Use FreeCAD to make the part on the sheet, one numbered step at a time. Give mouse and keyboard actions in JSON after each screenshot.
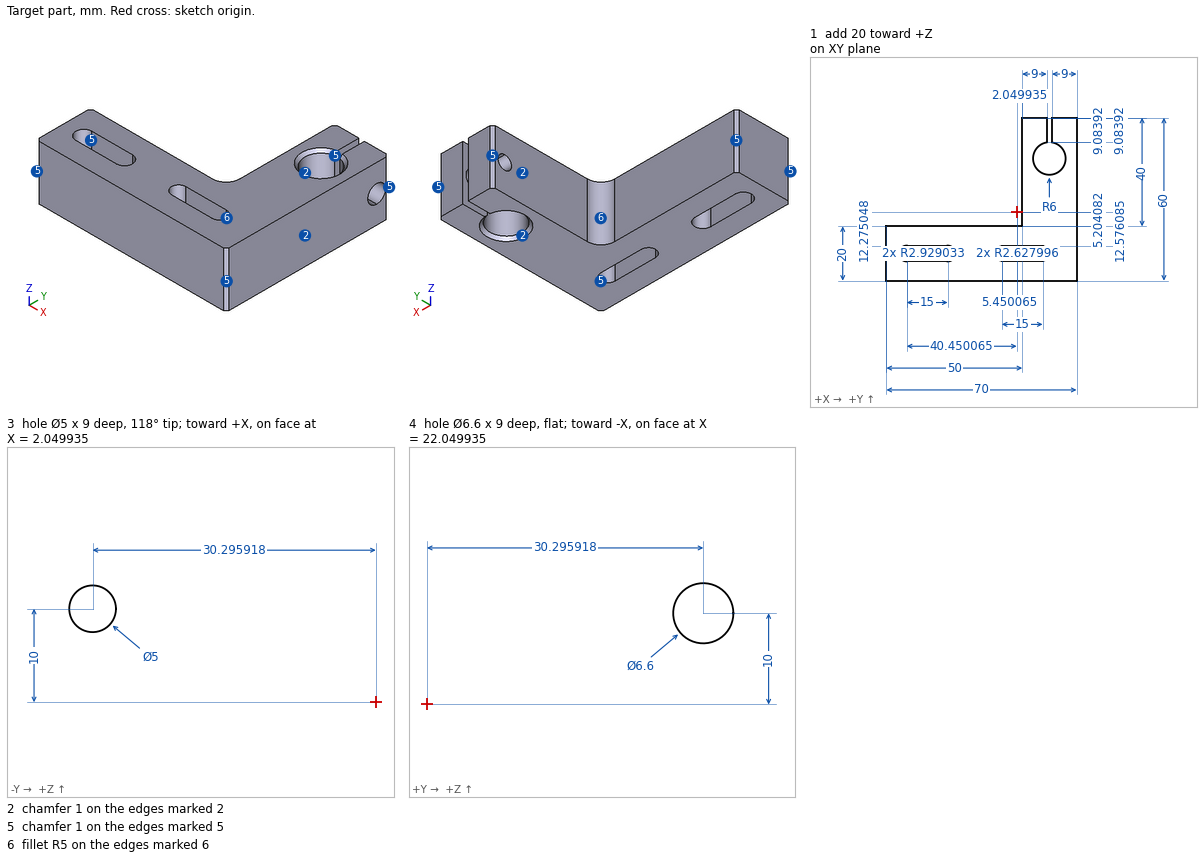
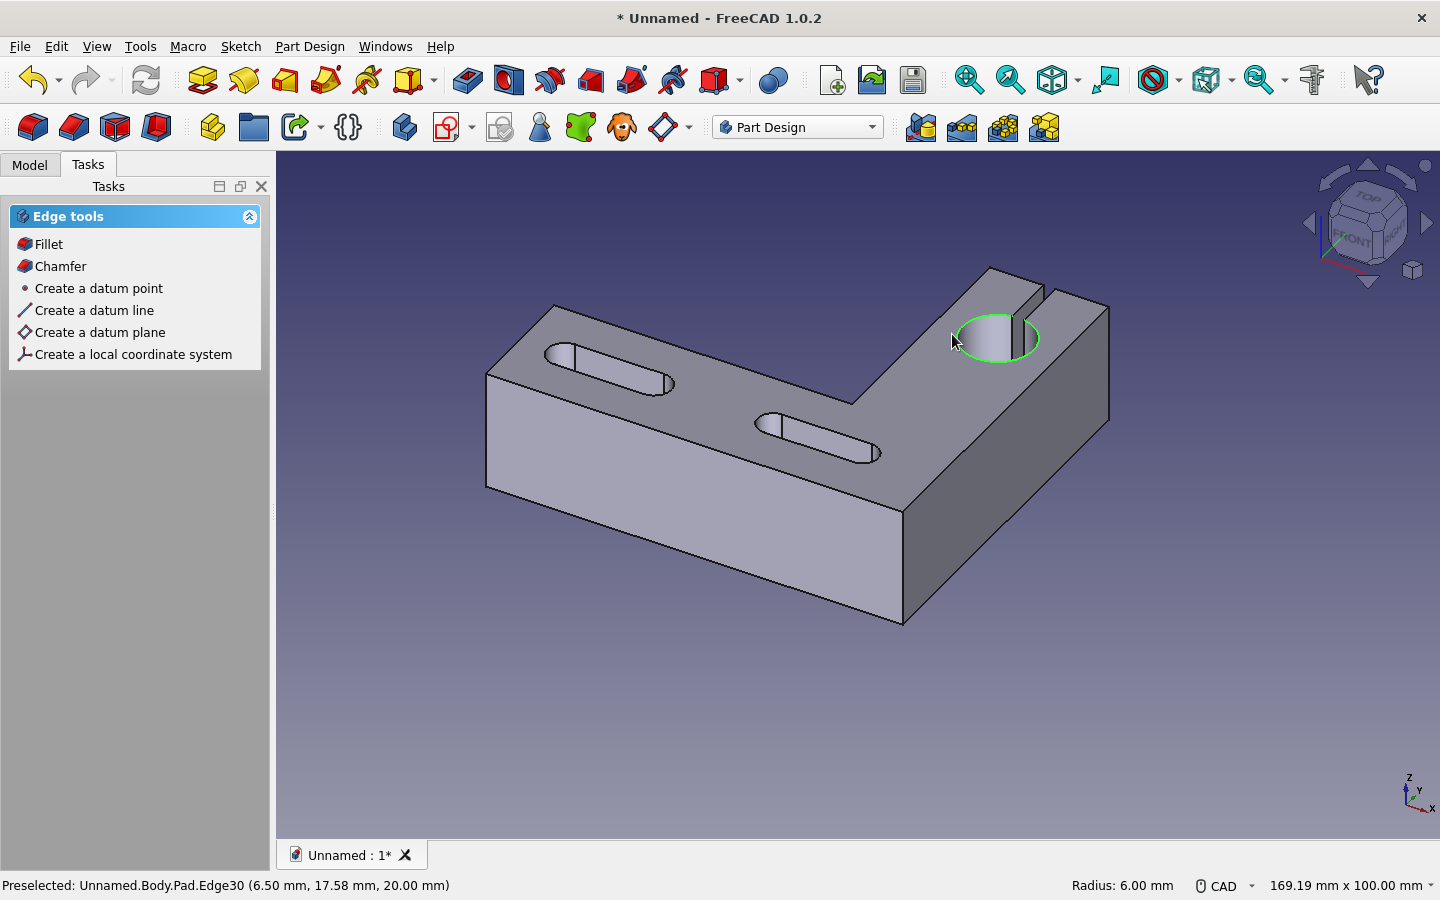
{"action": "key", "text": "0"}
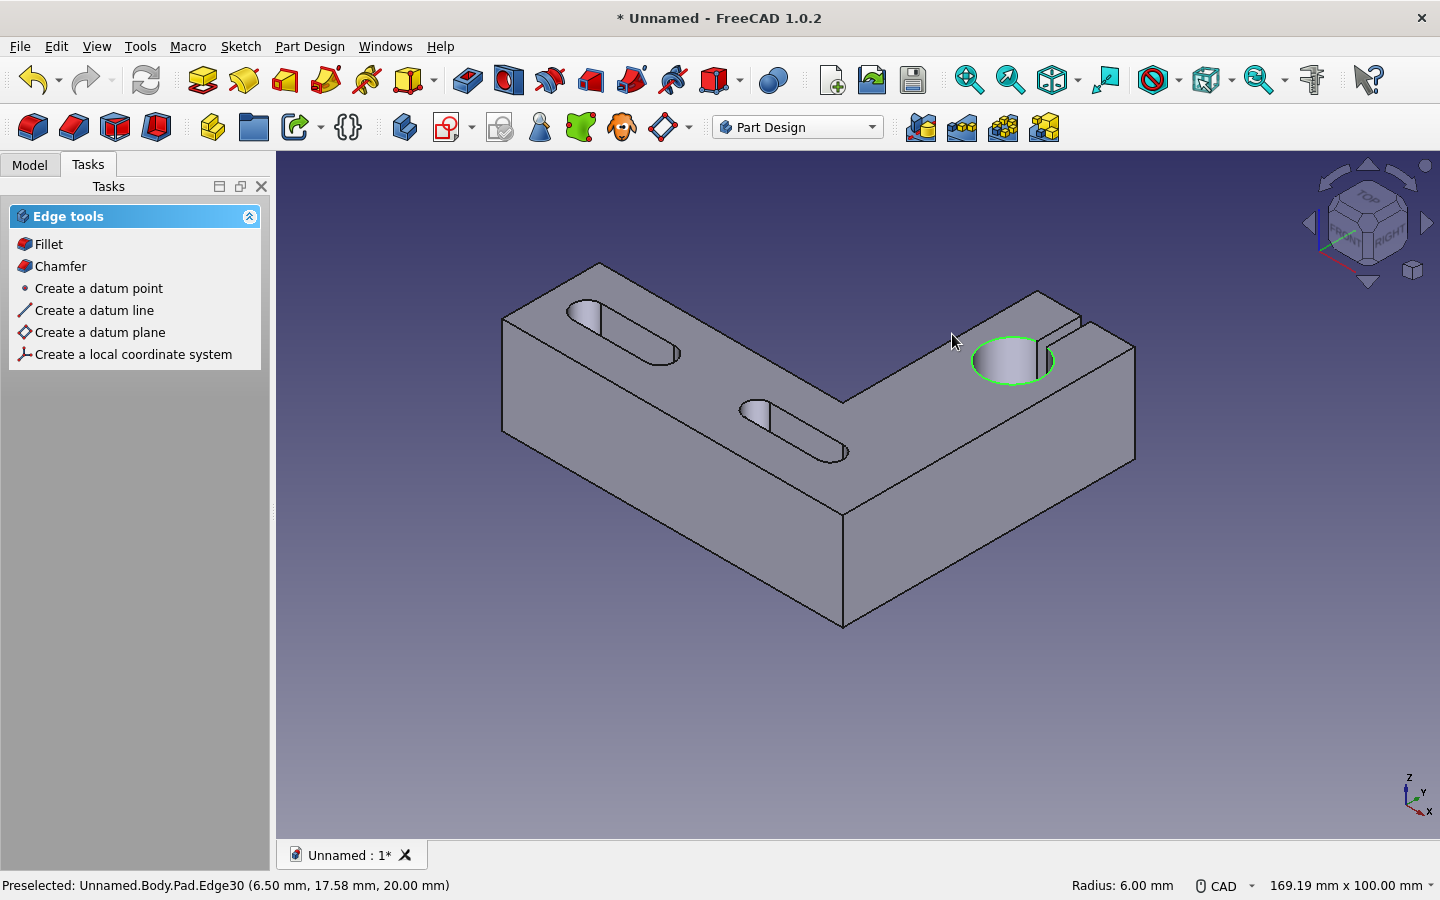
{"action": "left_click", "coordinate": [970, 80]}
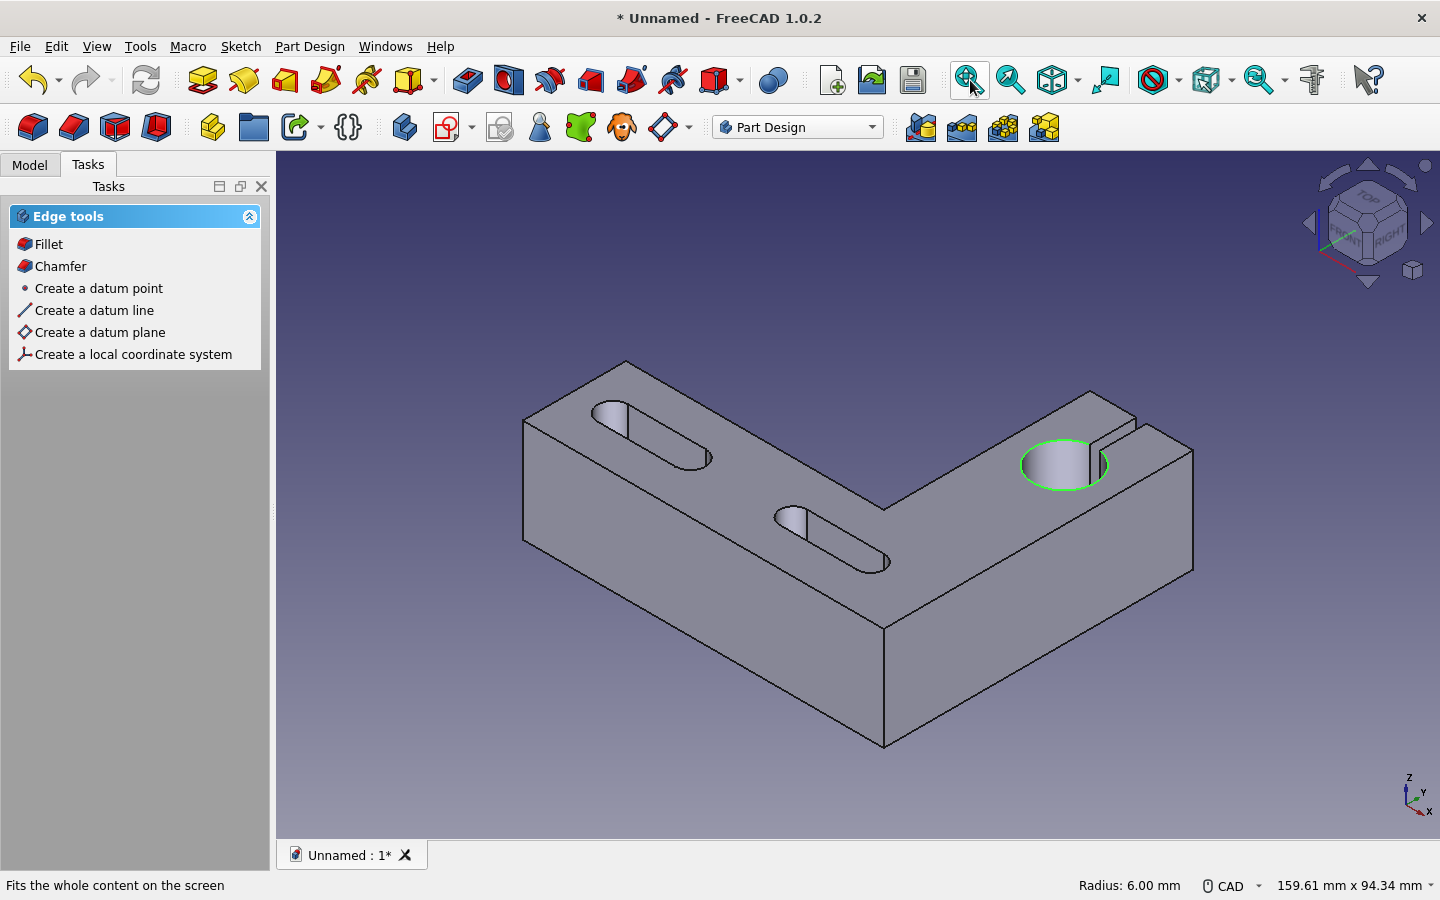
{"action": "key", "text": "2"}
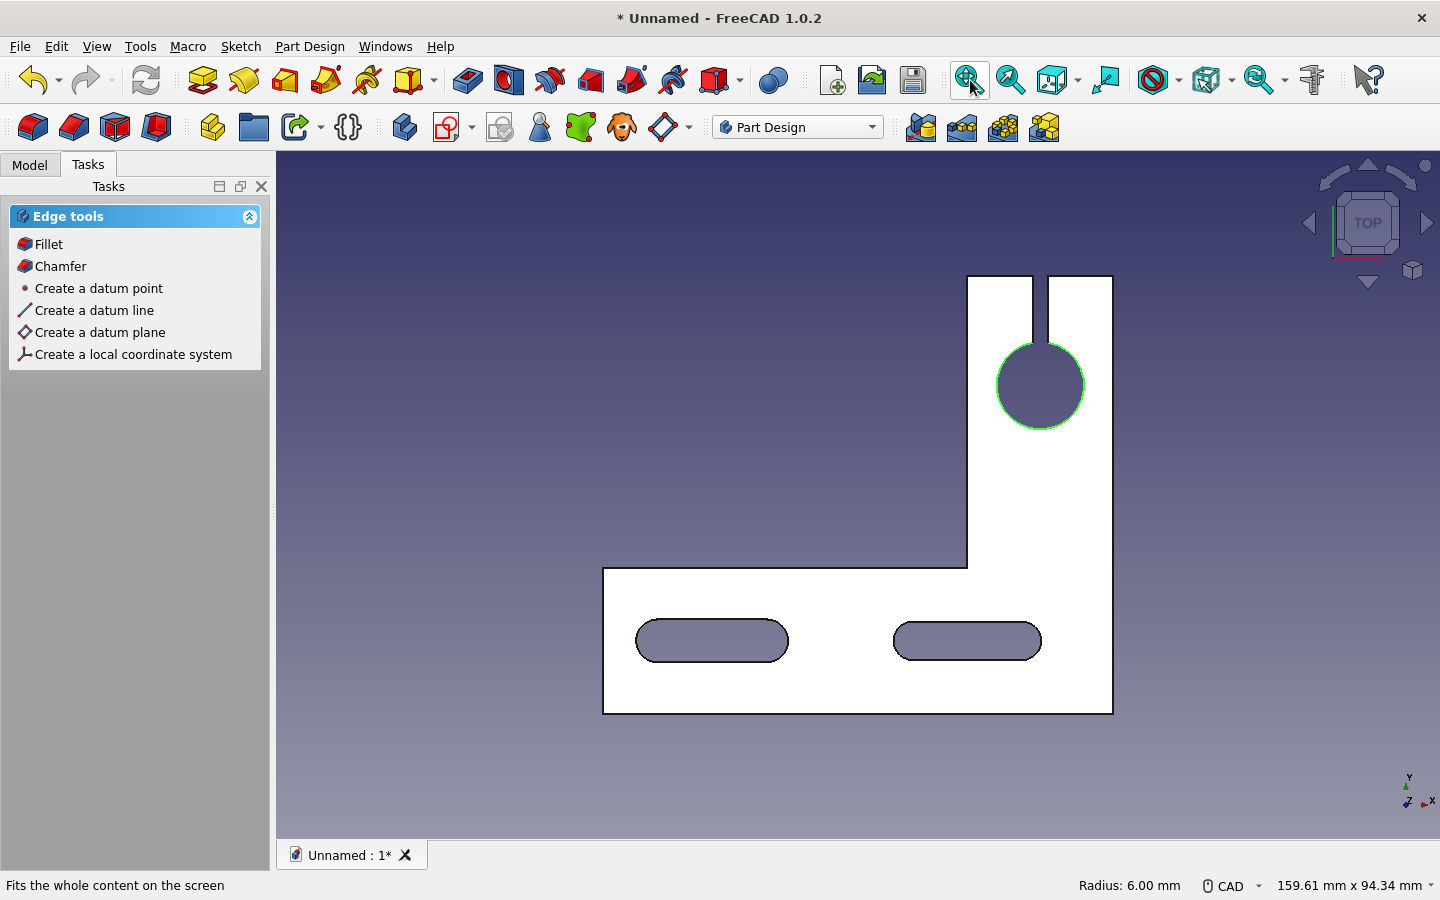
{"action": "key", "text": "1"}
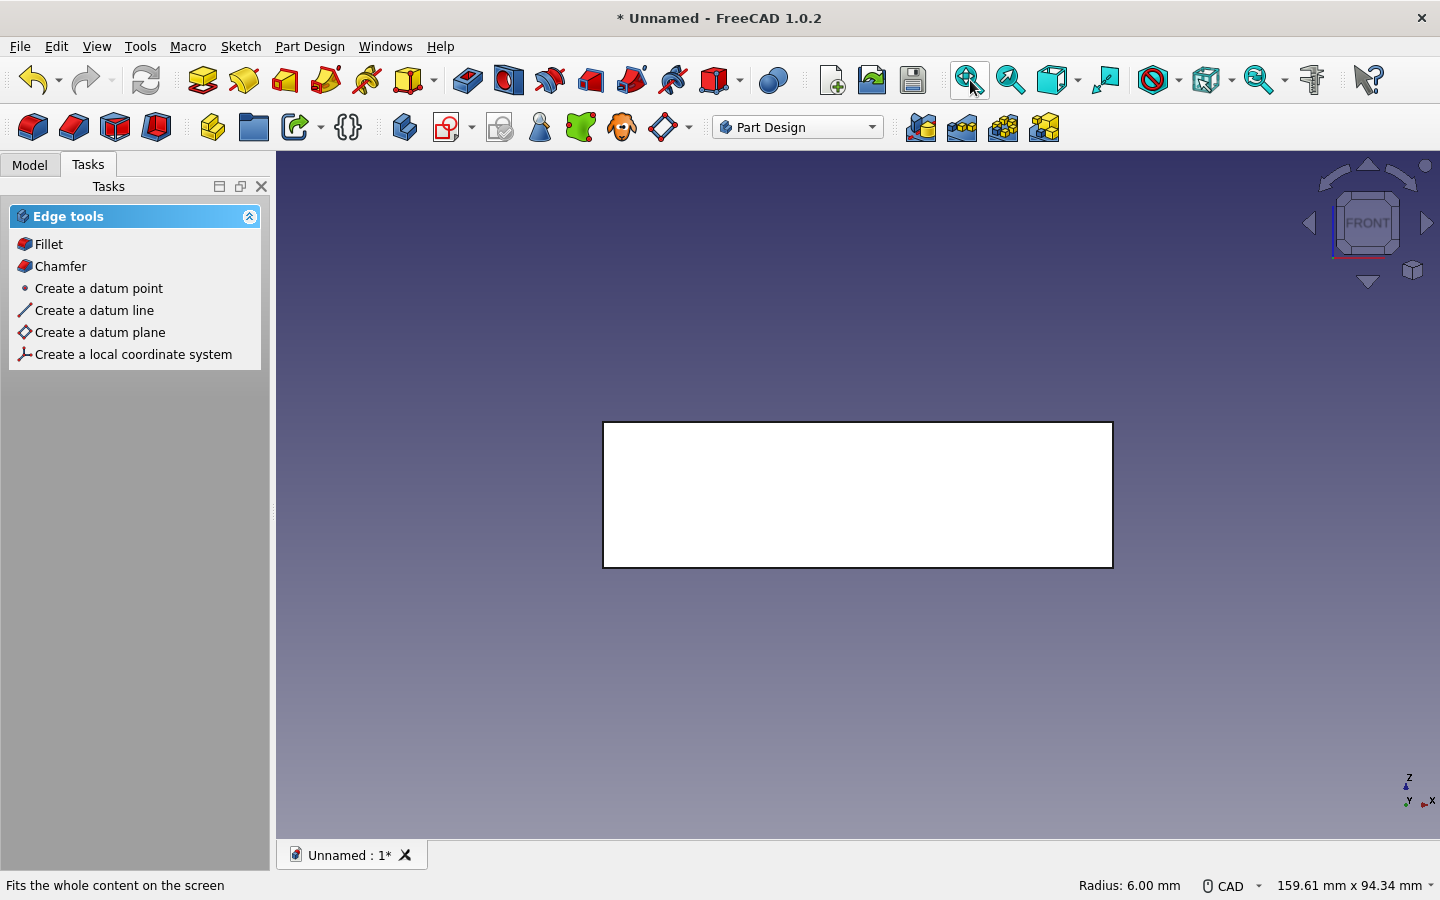
{"action": "left_click", "coordinate": [970, 80]}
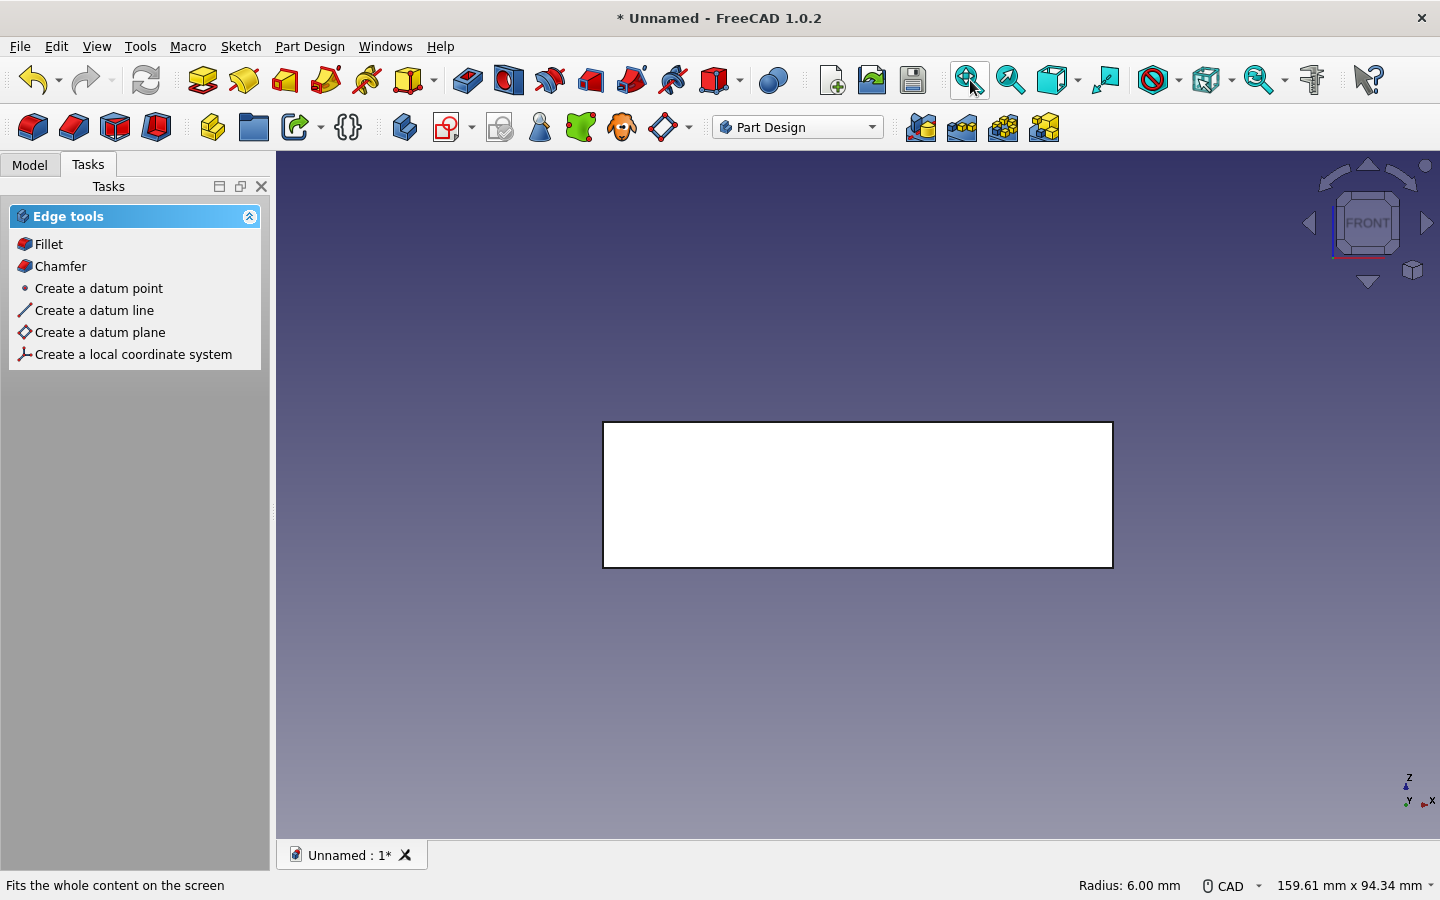
{"action": "key", "text": "3"}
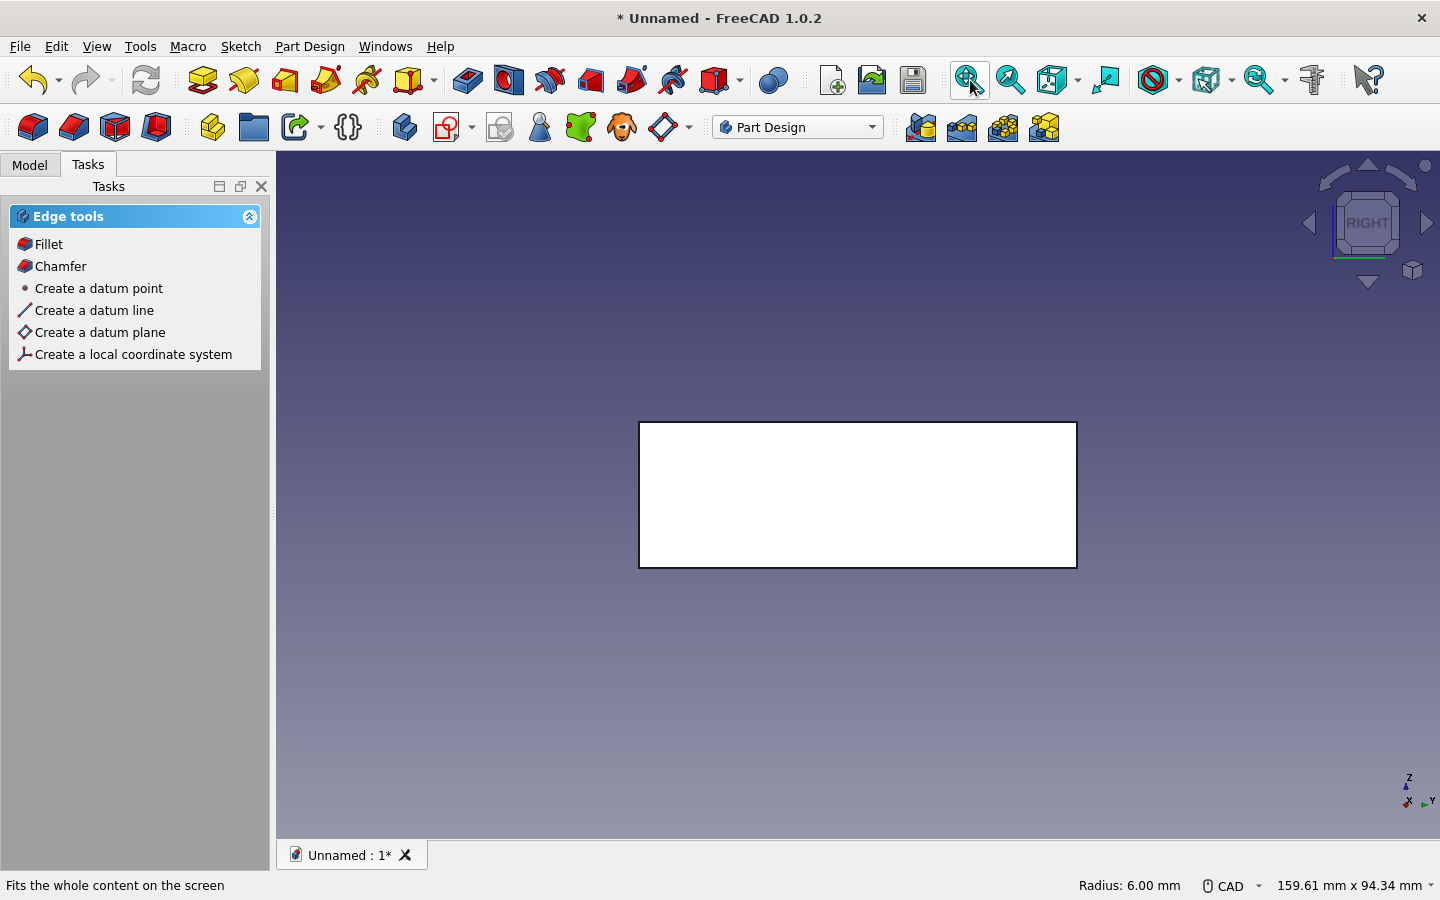
{"action": "left_click", "coordinate": [970, 80]}